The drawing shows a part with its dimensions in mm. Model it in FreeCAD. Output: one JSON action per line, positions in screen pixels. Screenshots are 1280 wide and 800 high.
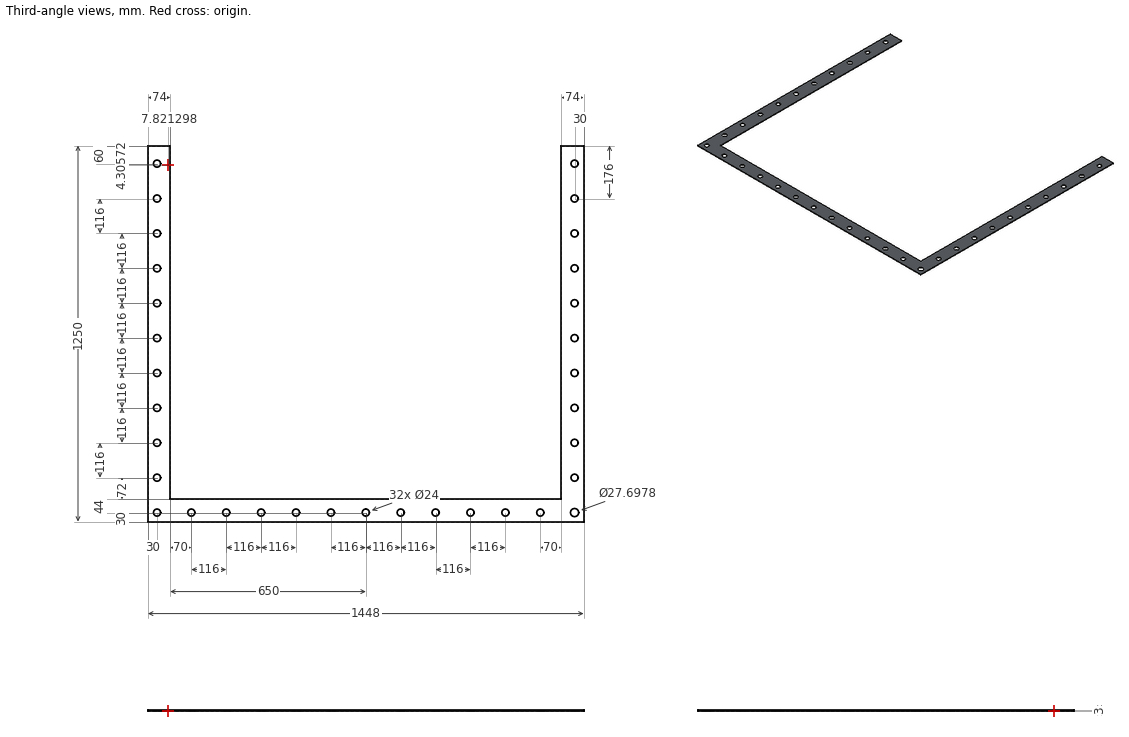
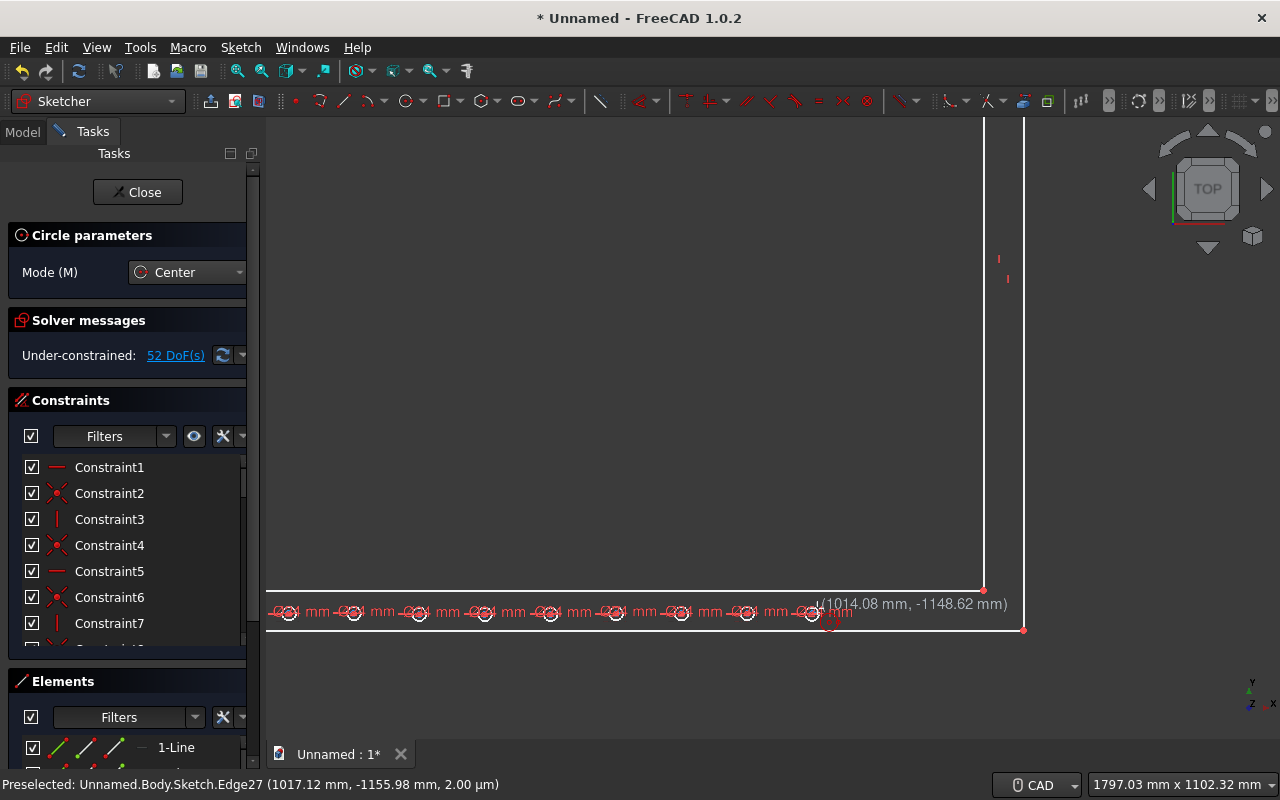
{"action": "scroll", "coordinate": [878, 613], "scroll_direction": "up", "scroll_amount": 7}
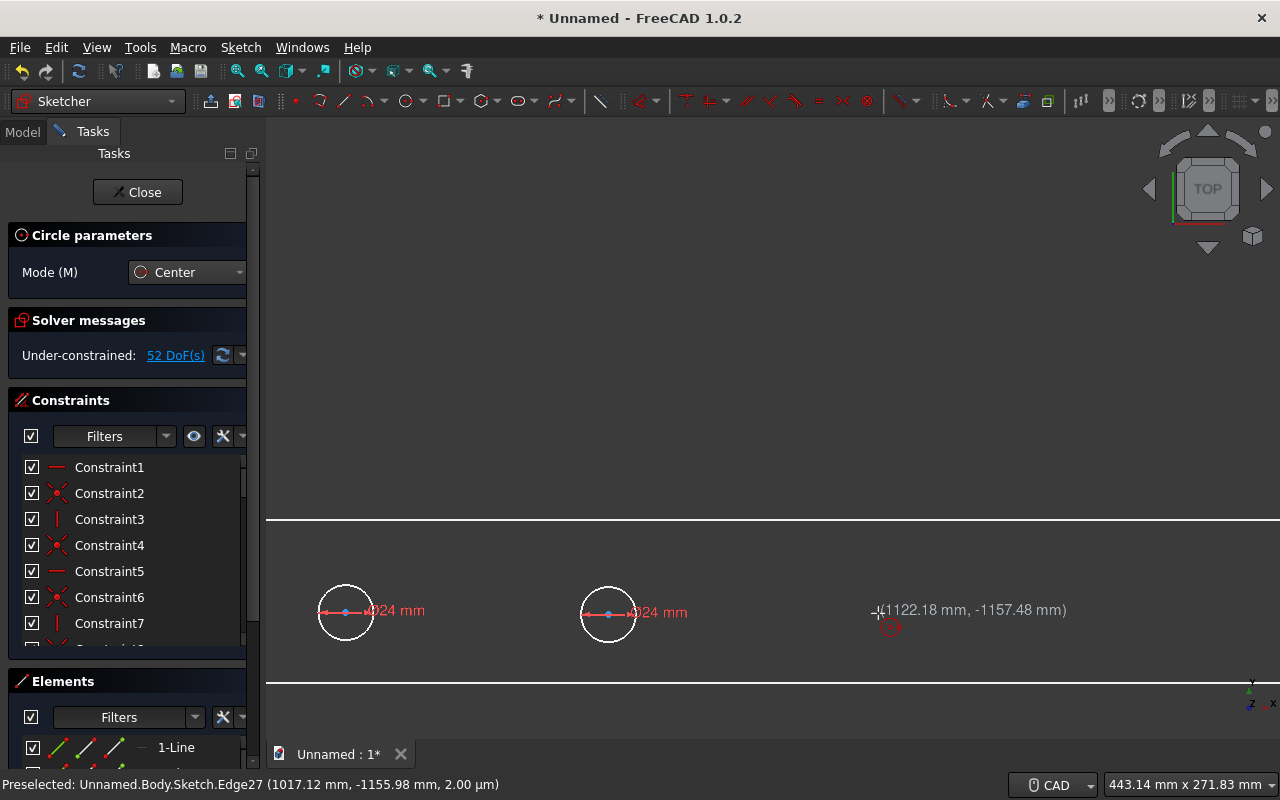
{"action": "scroll", "coordinate": [844, 613], "scroll_direction": "down", "scroll_amount": 10}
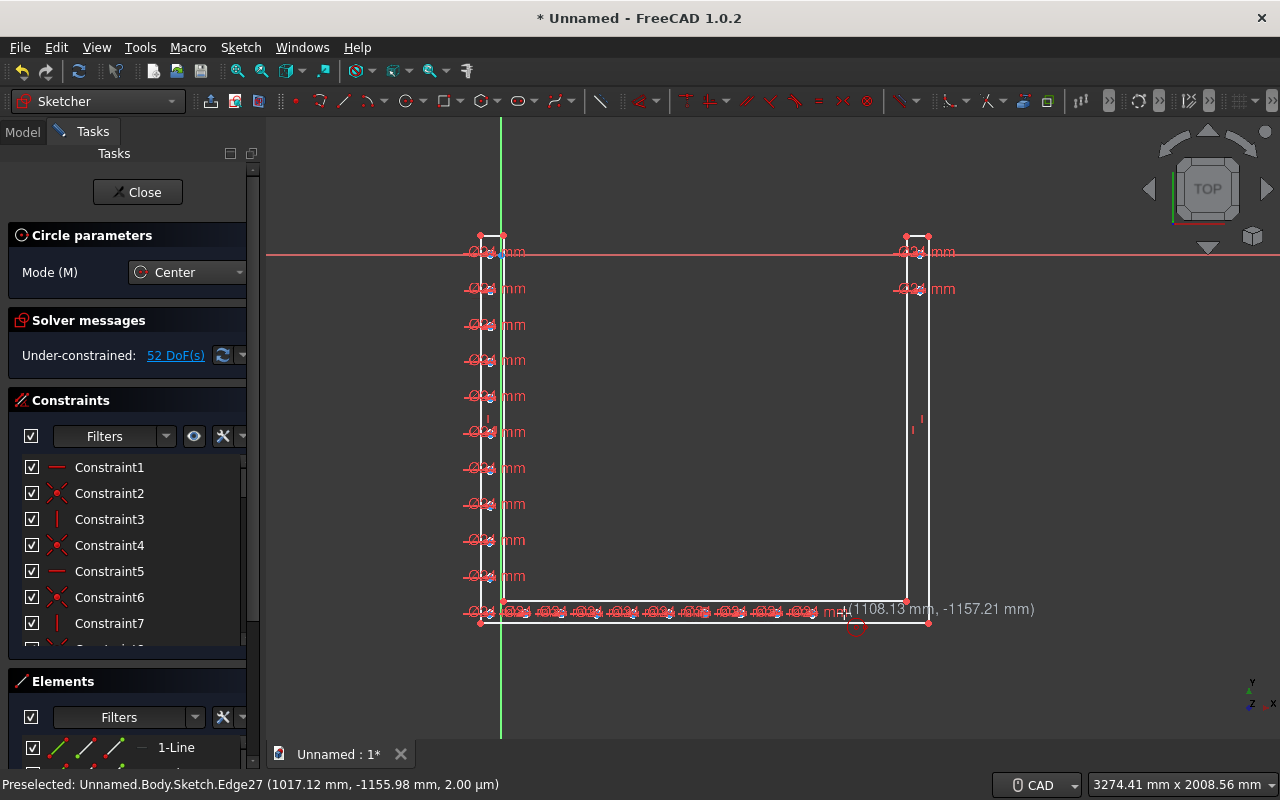
{"action": "scroll", "coordinate": [849, 613], "scroll_direction": "up", "scroll_amount": 3}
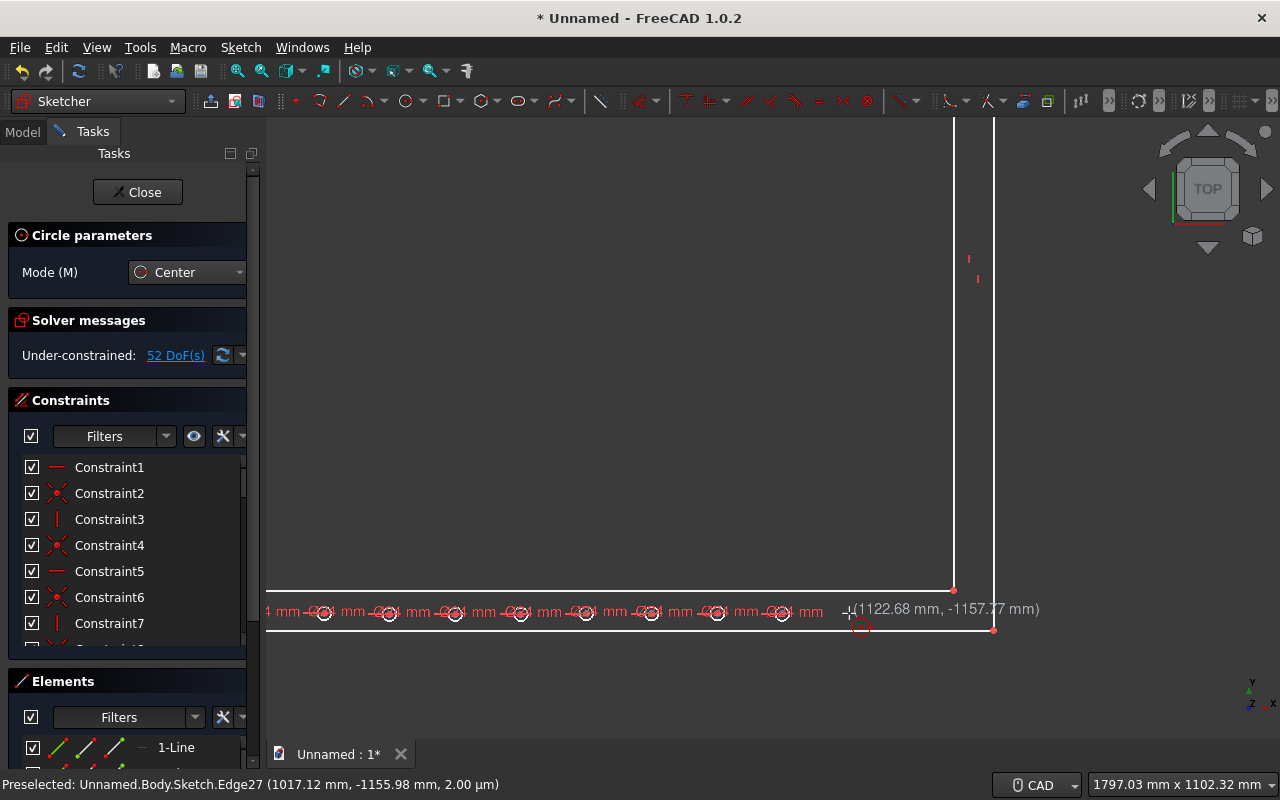
{"action": "left_click", "coordinate": [848, 613]}
{"action": "mouse_move", "coordinate": [853, 608]}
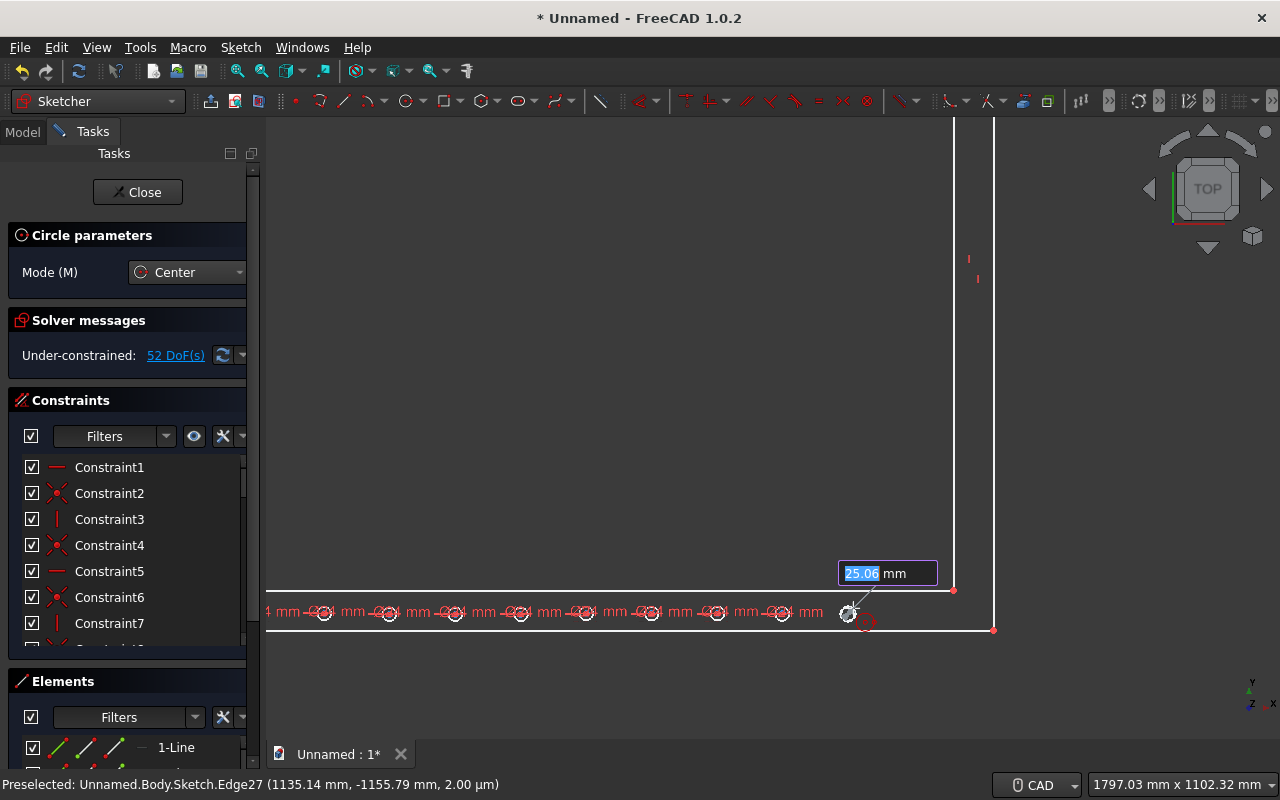
{"action": "type", "text": "24"}
{"action": "key", "text": "Return"}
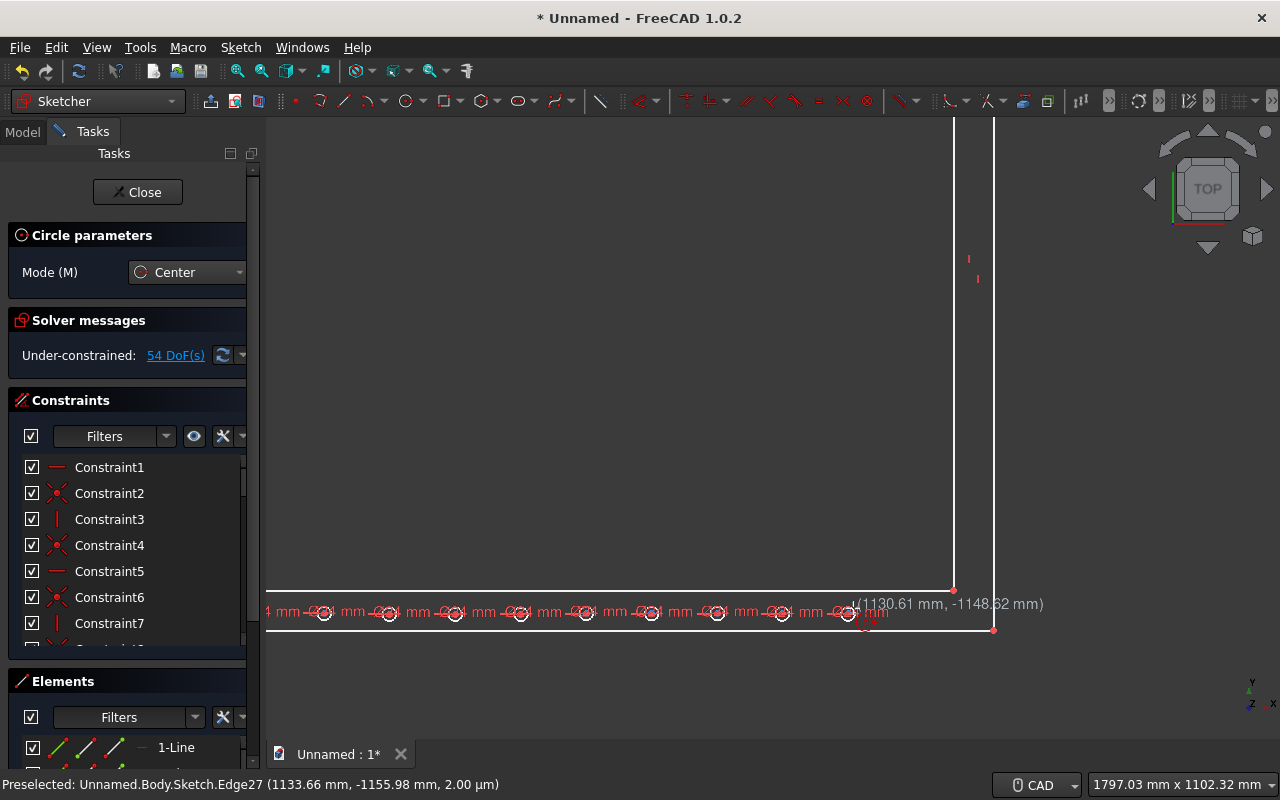
{"action": "scroll", "coordinate": [913, 613], "scroll_direction": "up", "scroll_amount": 7}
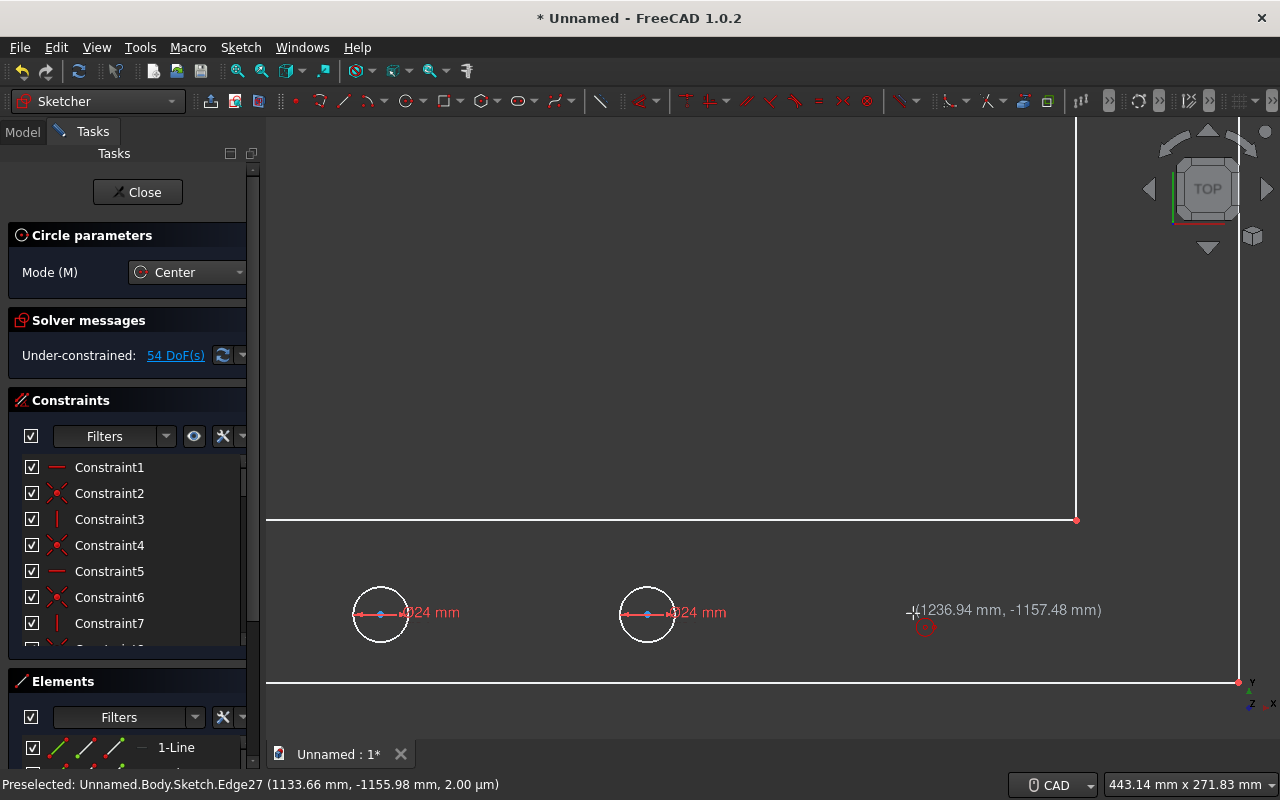
{"action": "scroll", "coordinate": [880, 613], "scroll_direction": "down", "scroll_amount": 10}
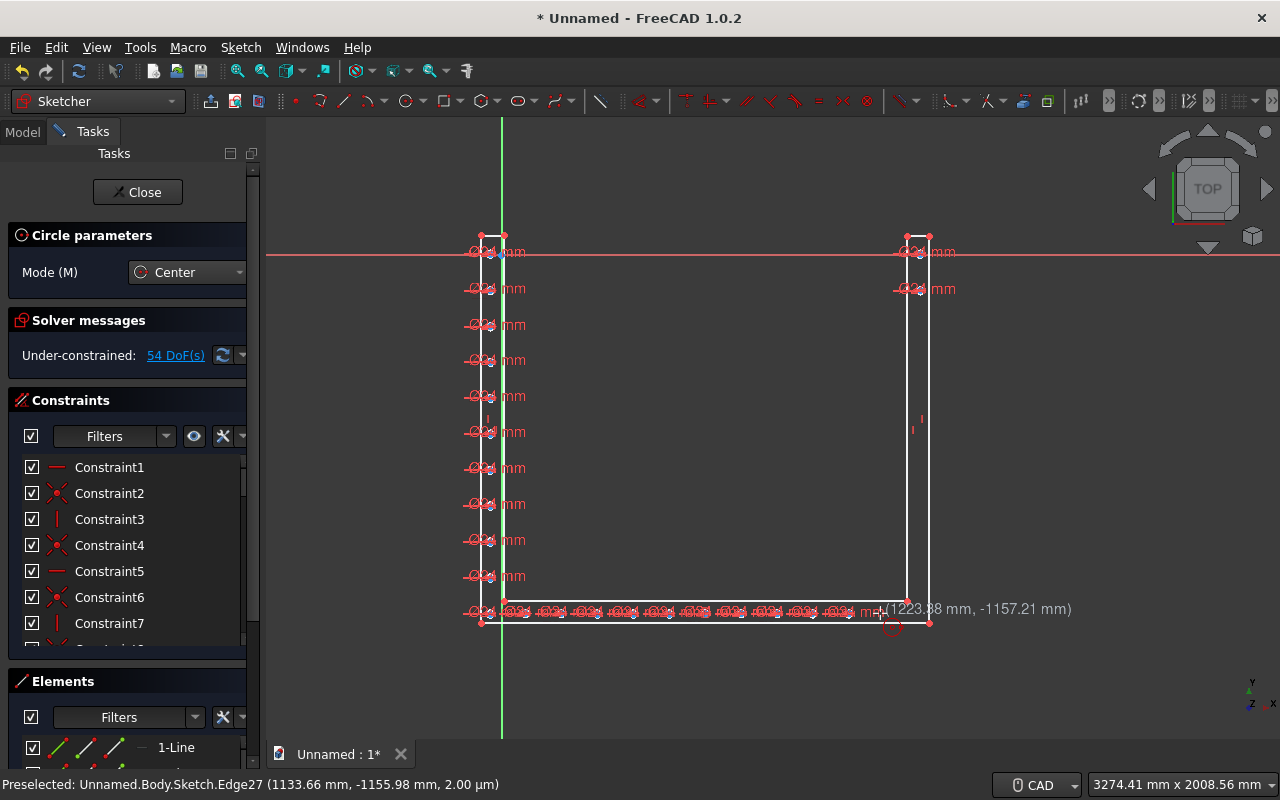
{"action": "scroll", "coordinate": [885, 613], "scroll_direction": "up", "scroll_amount": 3}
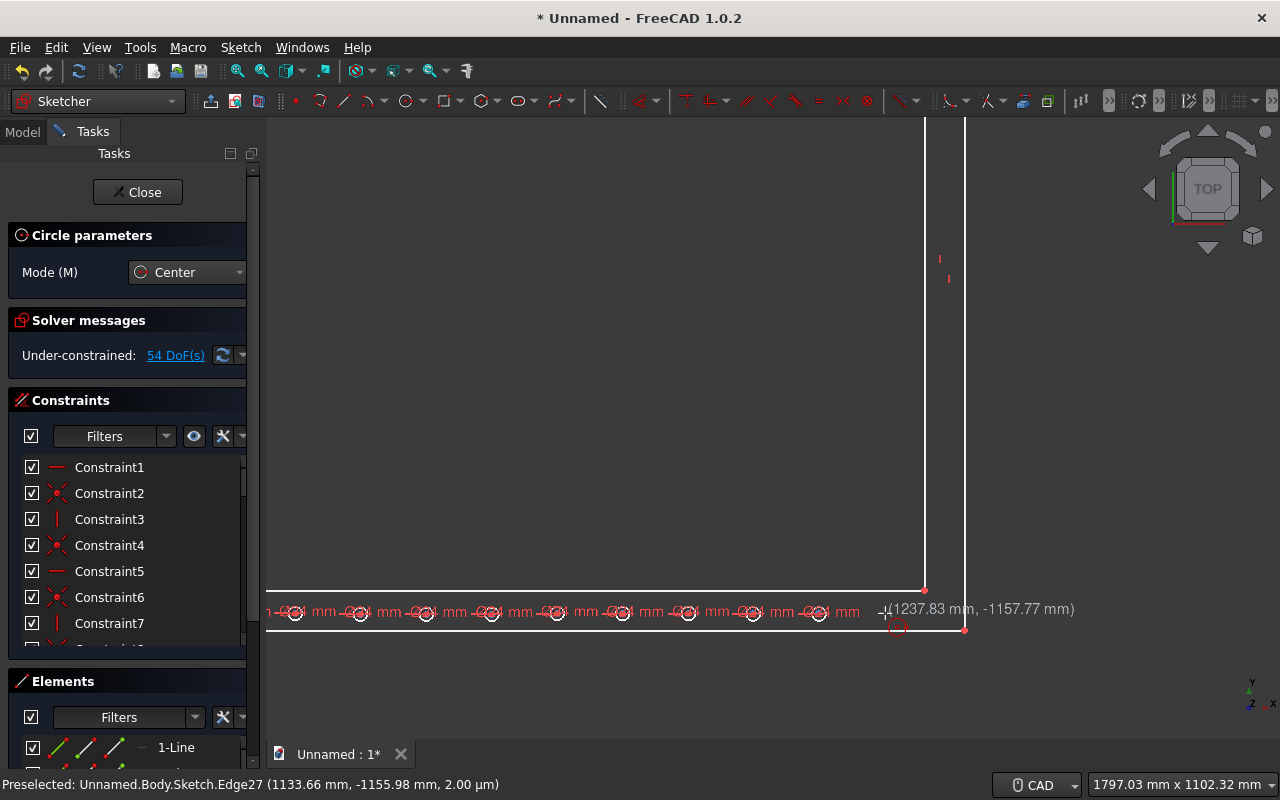
{"action": "left_click", "coordinate": [884, 613]}
{"action": "mouse_move", "coordinate": [889, 608]}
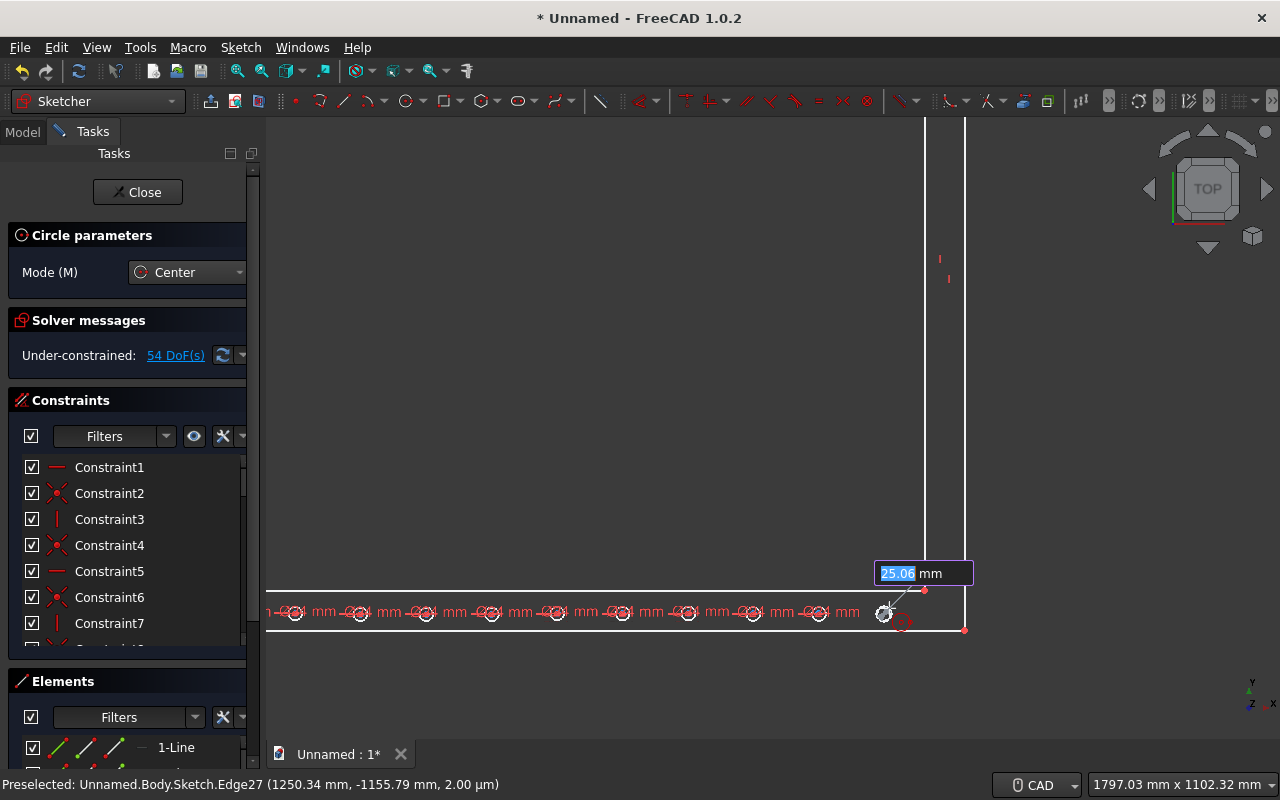
{"action": "type", "text": "24"}
{"action": "key", "text": "Return"}